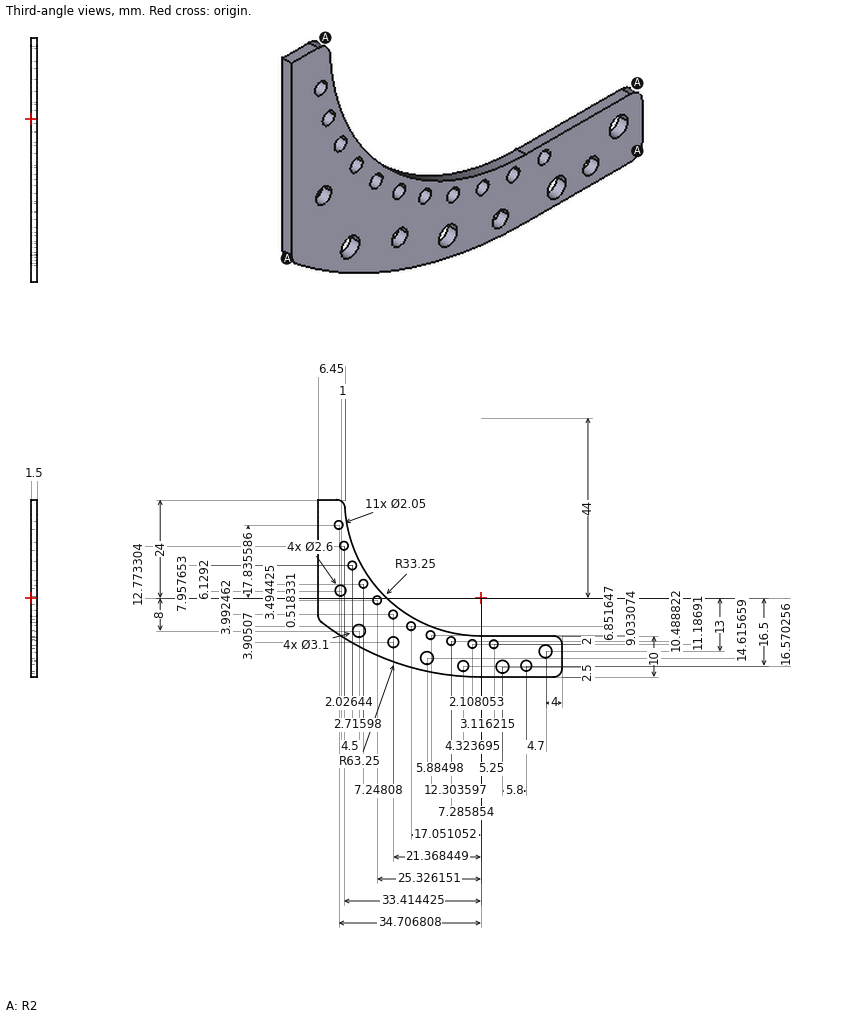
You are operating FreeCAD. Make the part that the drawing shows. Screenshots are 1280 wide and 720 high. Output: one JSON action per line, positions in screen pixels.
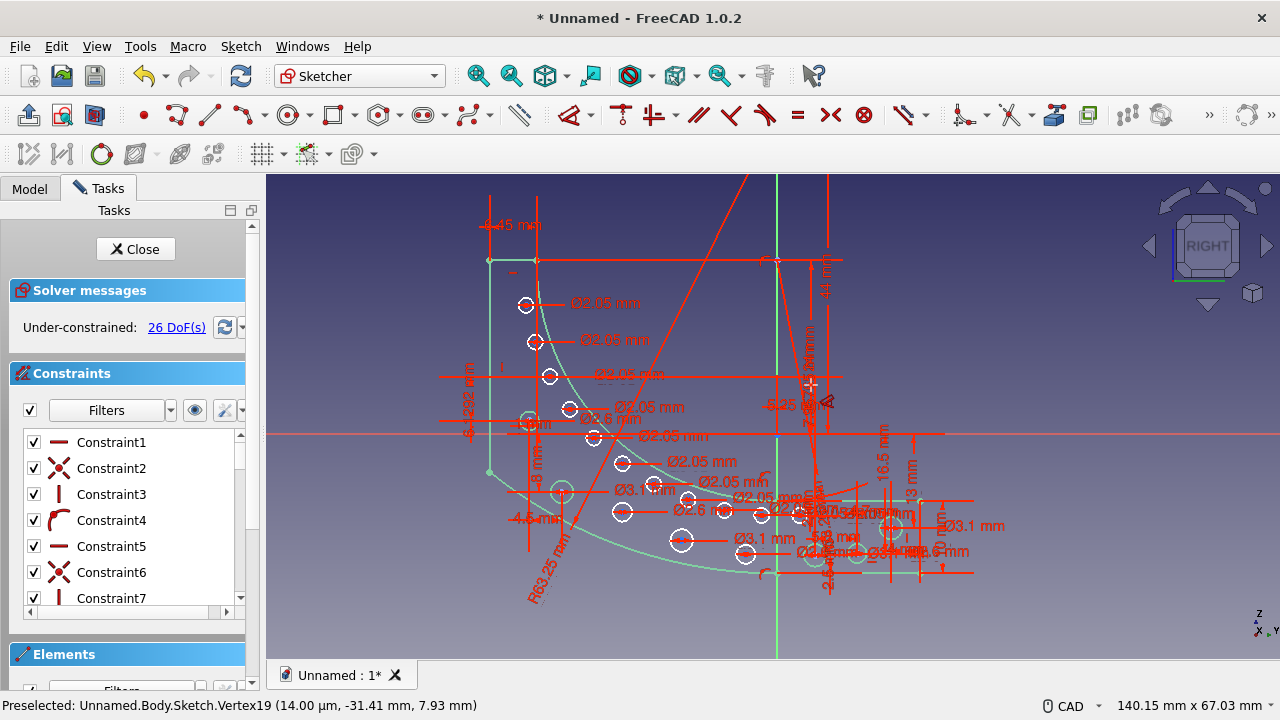
{"action": "scroll", "coordinate": [570, 409], "scroll_direction": "up", "scroll_amount": 3}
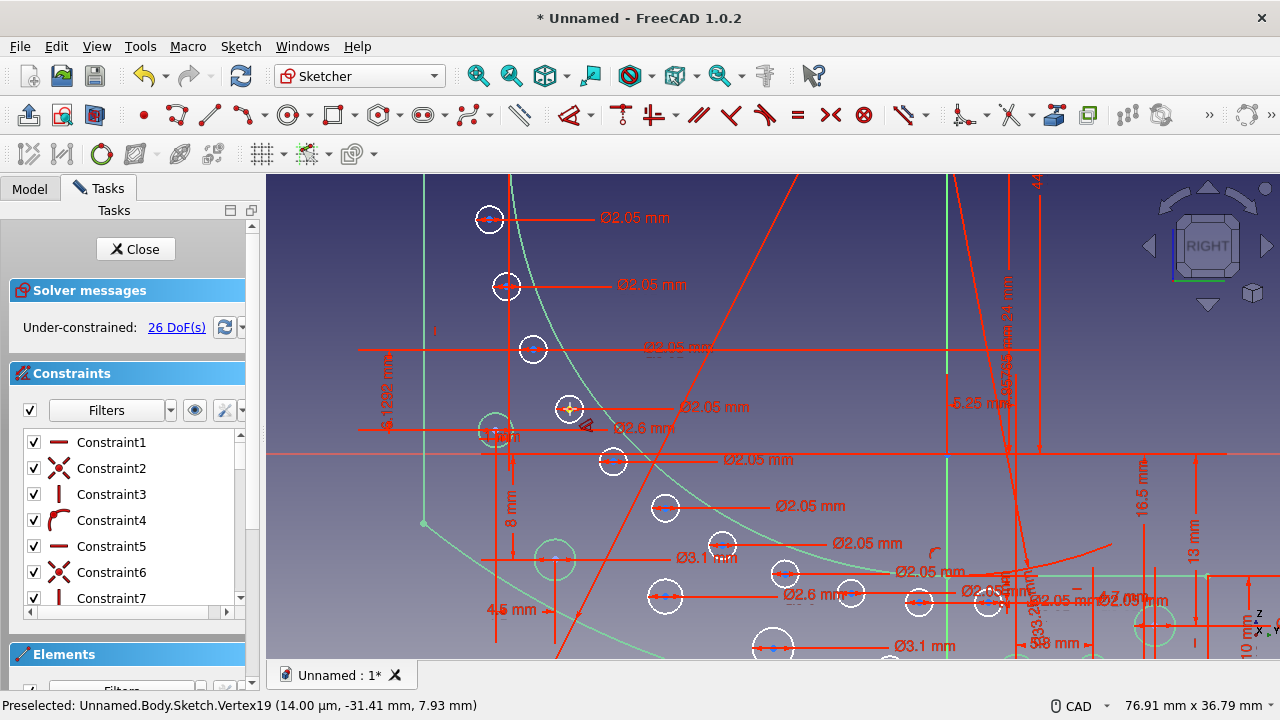
{"action": "left_click", "coordinate": [570, 409]}
{"action": "left_click", "coordinate": [536, 416]}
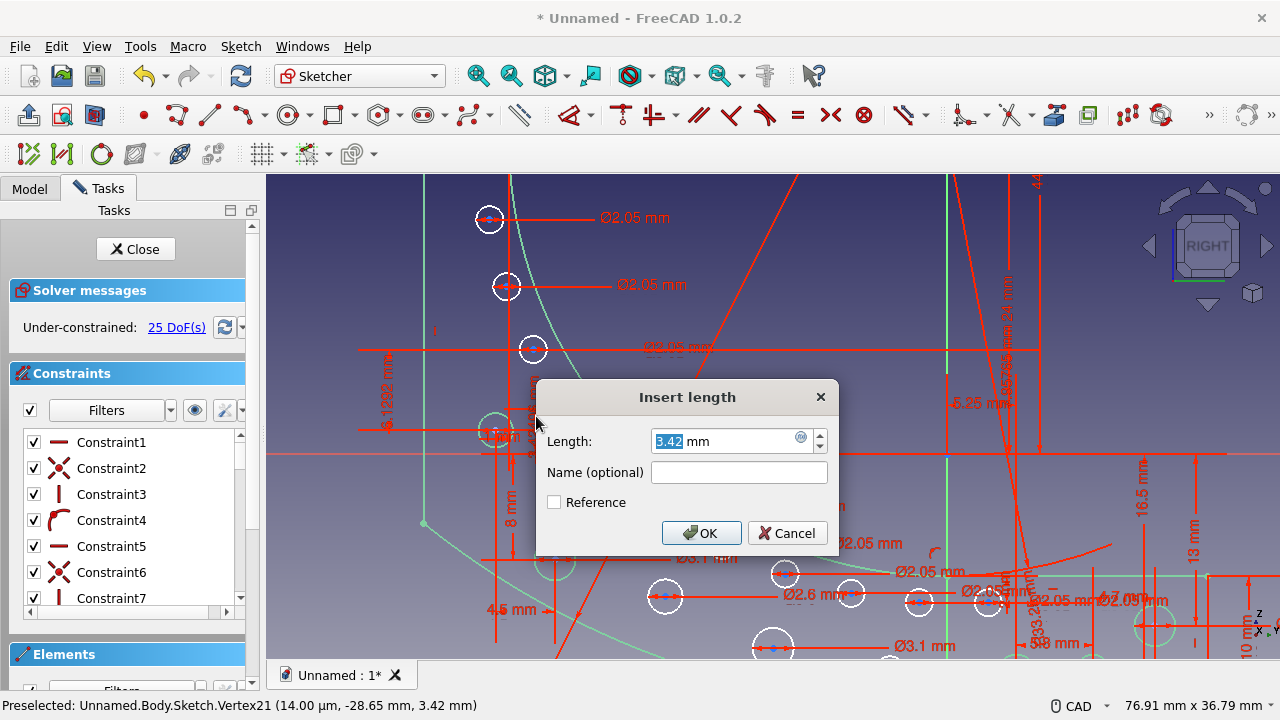
{"action": "type", "text": "3.494425"}
{"action": "key", "text": "Return"}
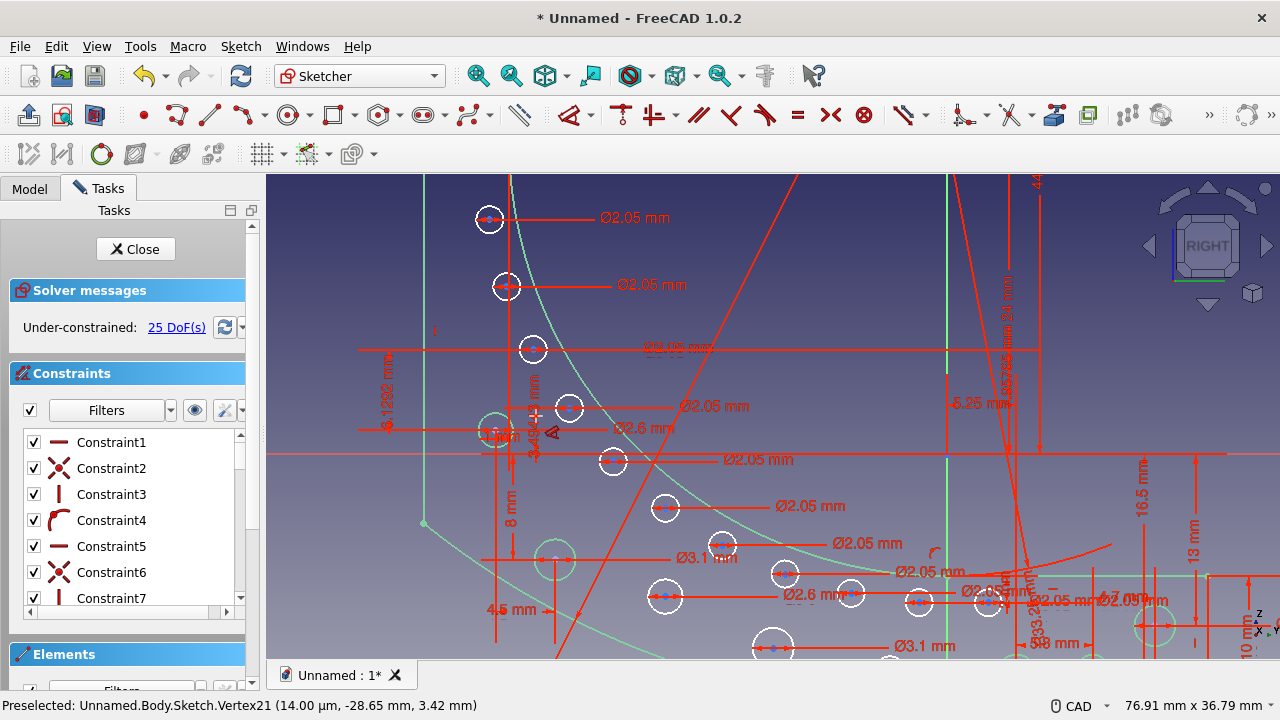
{"action": "scroll", "coordinate": [613, 462], "scroll_direction": "up", "scroll_amount": 9}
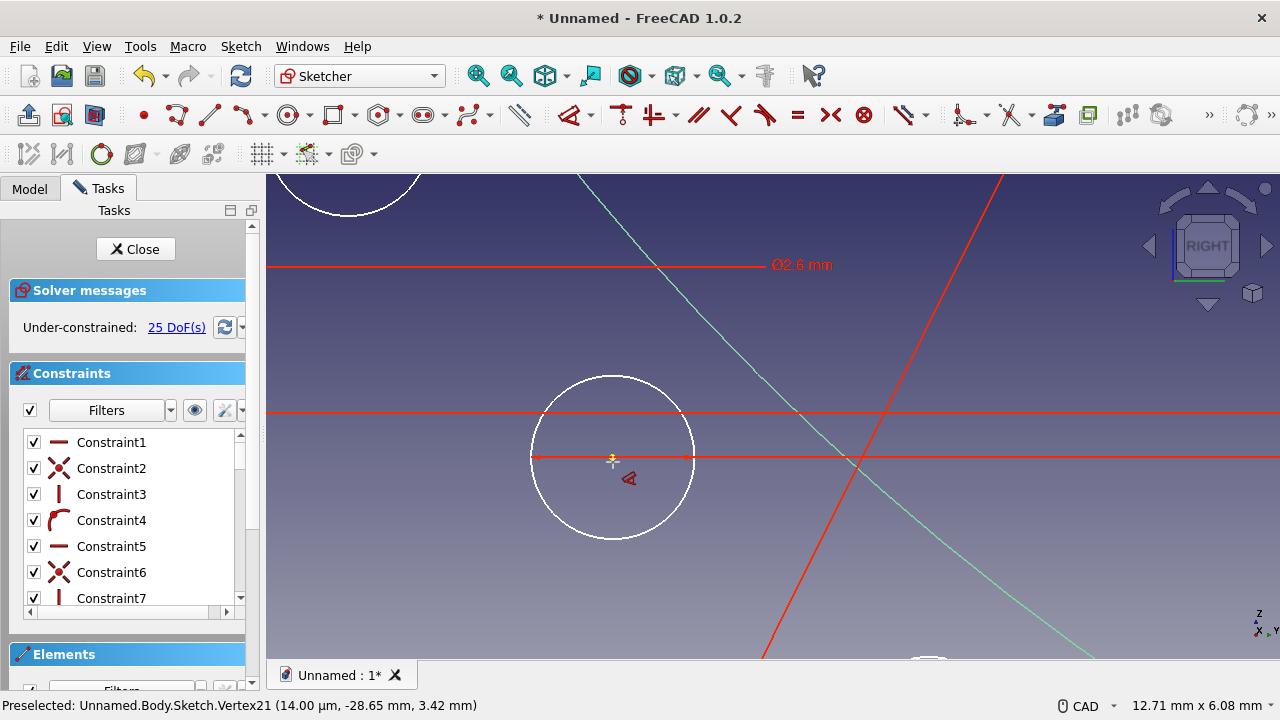
{"action": "left_click", "coordinate": [613, 457]}
{"action": "left_click", "coordinate": [579, 435]}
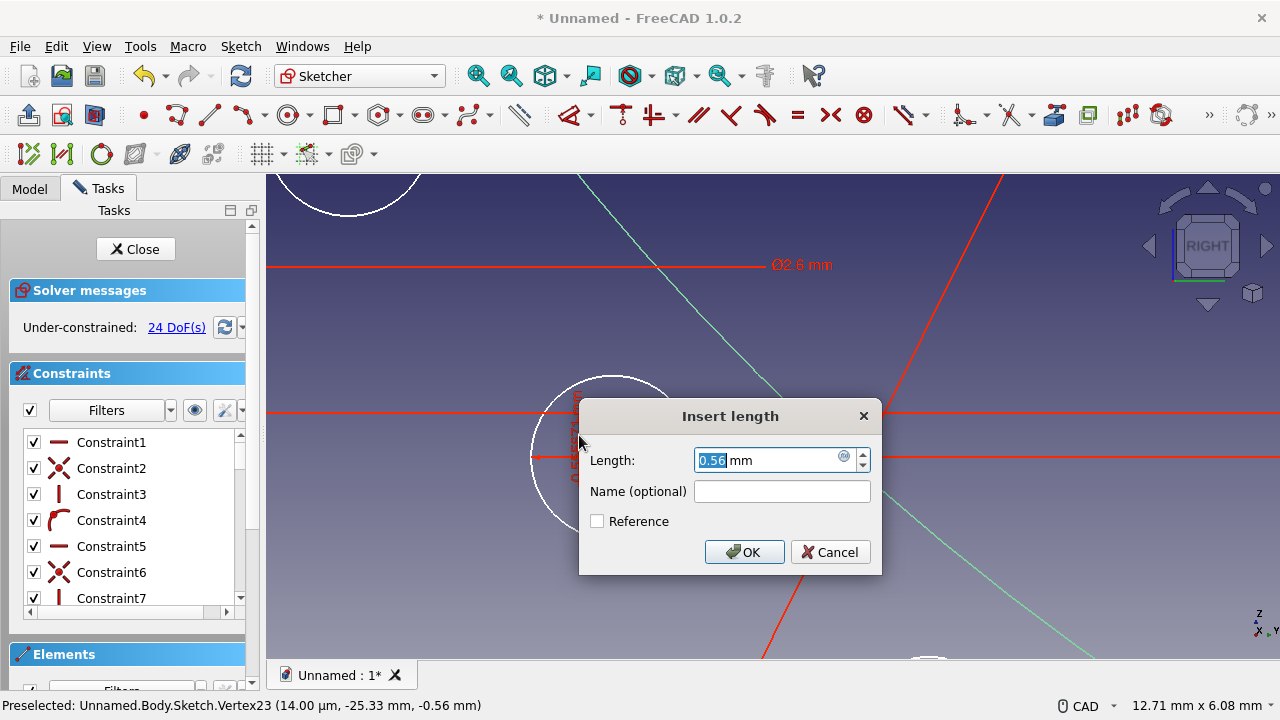
{"action": "type", "text": "0.518331"}
{"action": "key", "text": "Return"}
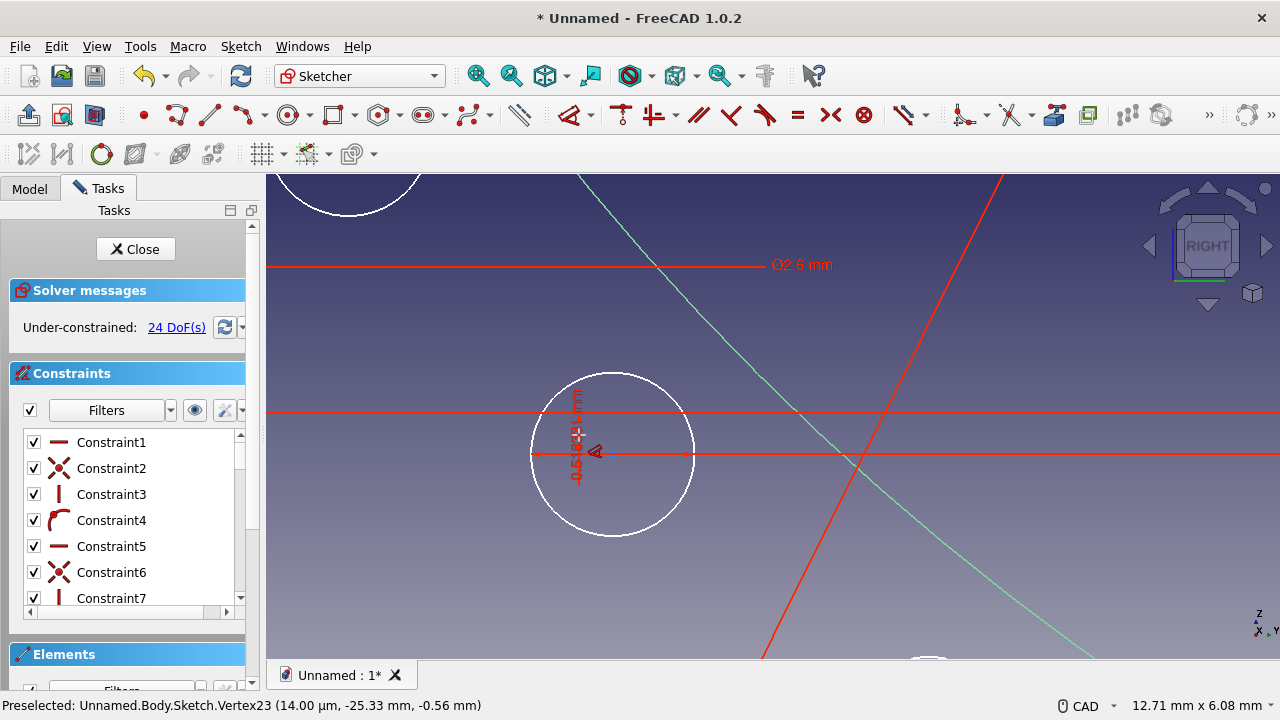
{"action": "scroll", "coordinate": [591, 436], "scroll_direction": "down", "scroll_amount": 12}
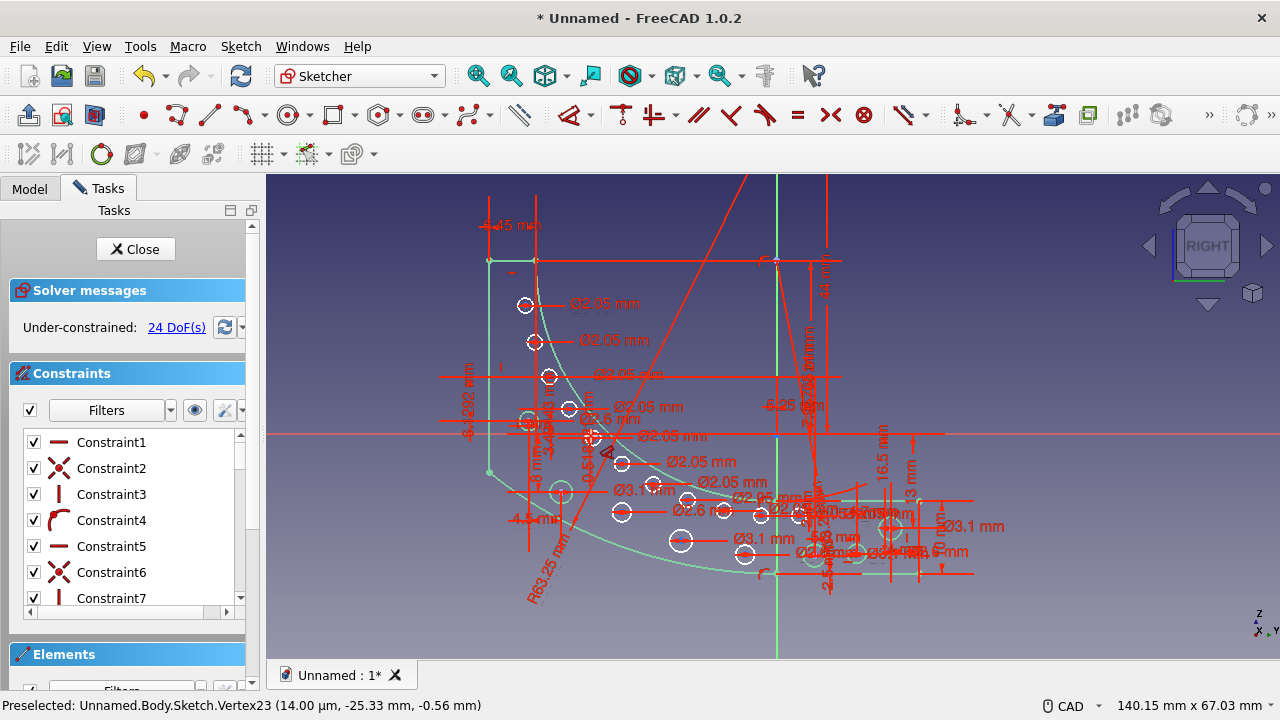
{"action": "scroll", "coordinate": [622, 464], "scroll_direction": "up", "scroll_amount": 2}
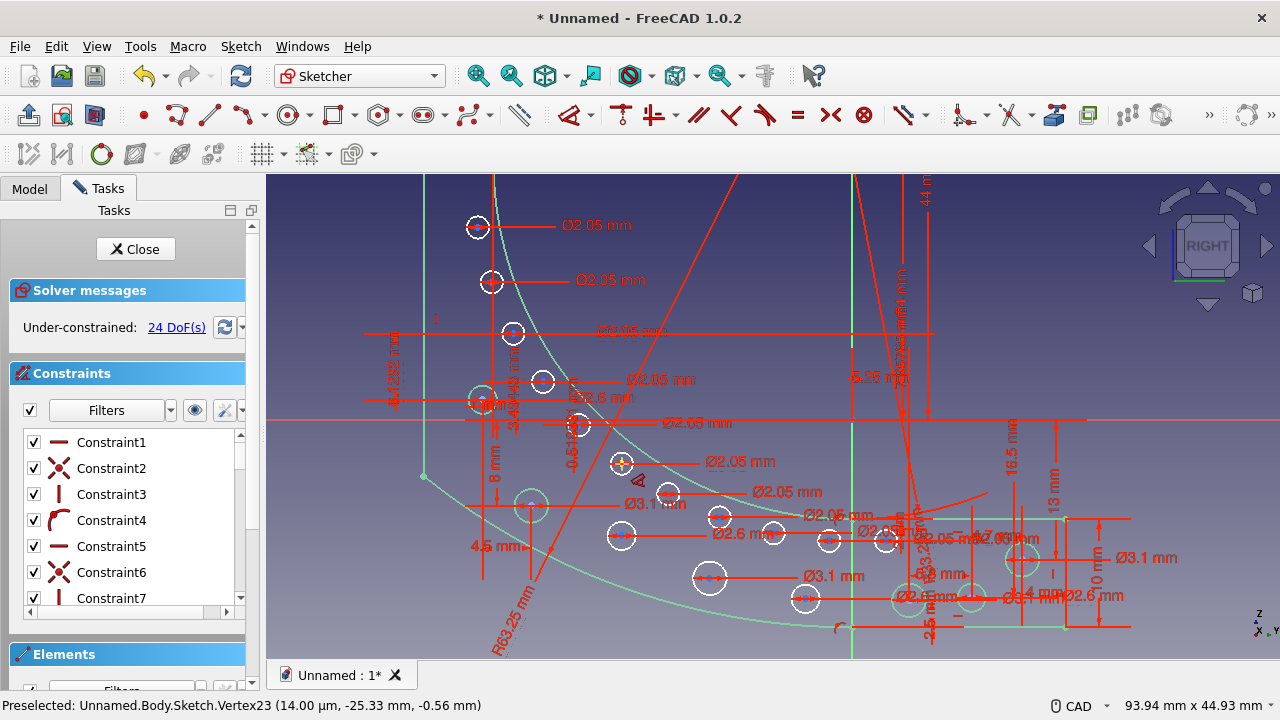
{"action": "left_click", "coordinate": [622, 464]}
{"action": "left_click", "coordinate": [588, 452]}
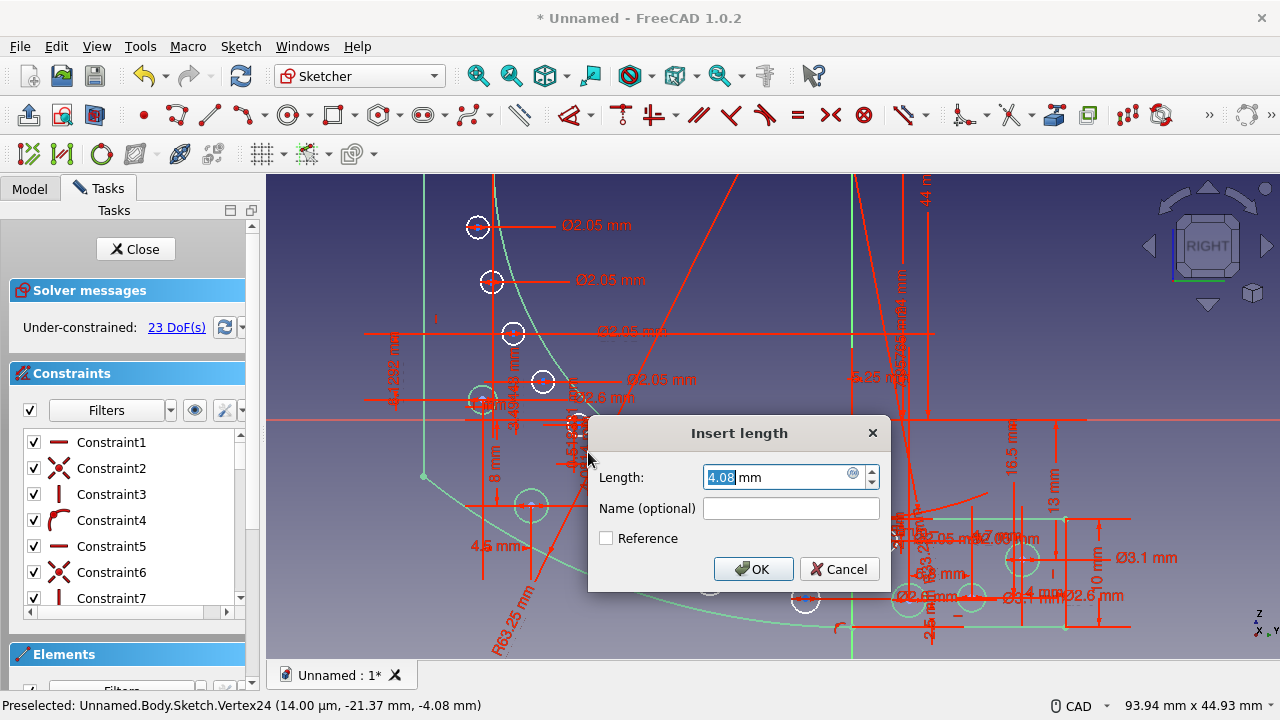
{"action": "type", "text": "3.992462"}
{"action": "key", "text": "Return"}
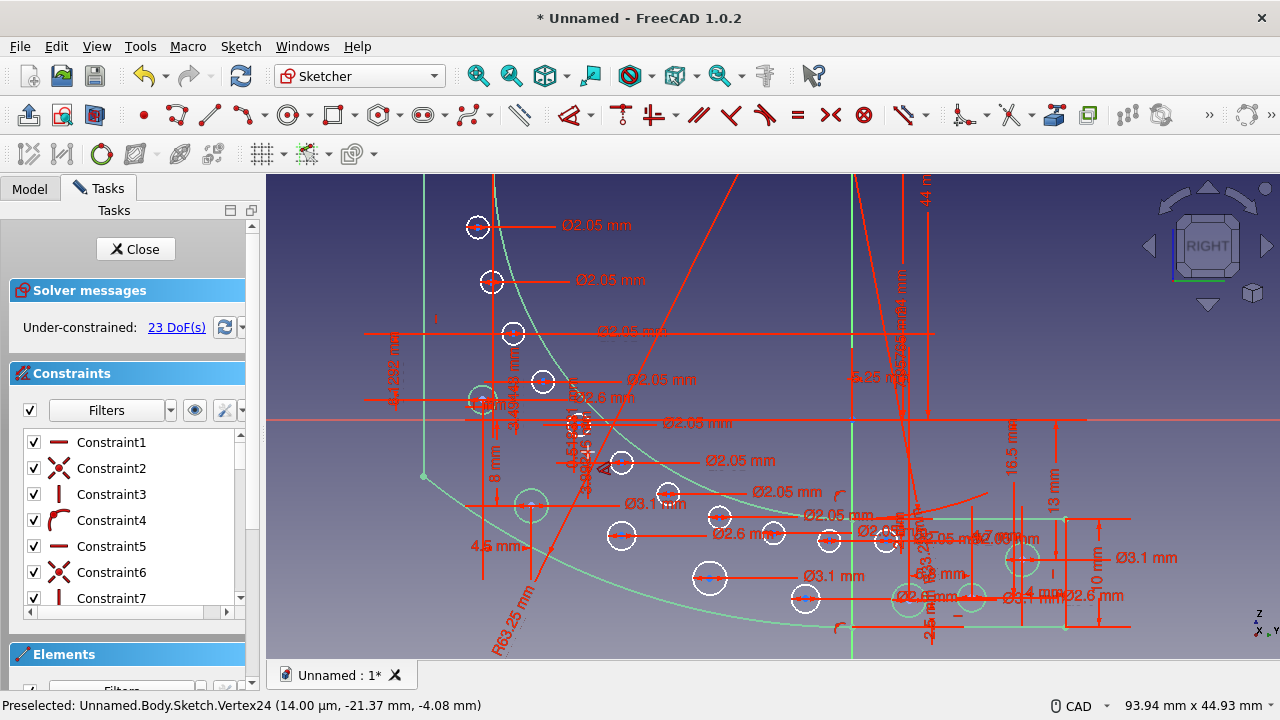
{"action": "left_click", "coordinate": [668, 494]}
{"action": "left_click", "coordinate": [886, 457]}